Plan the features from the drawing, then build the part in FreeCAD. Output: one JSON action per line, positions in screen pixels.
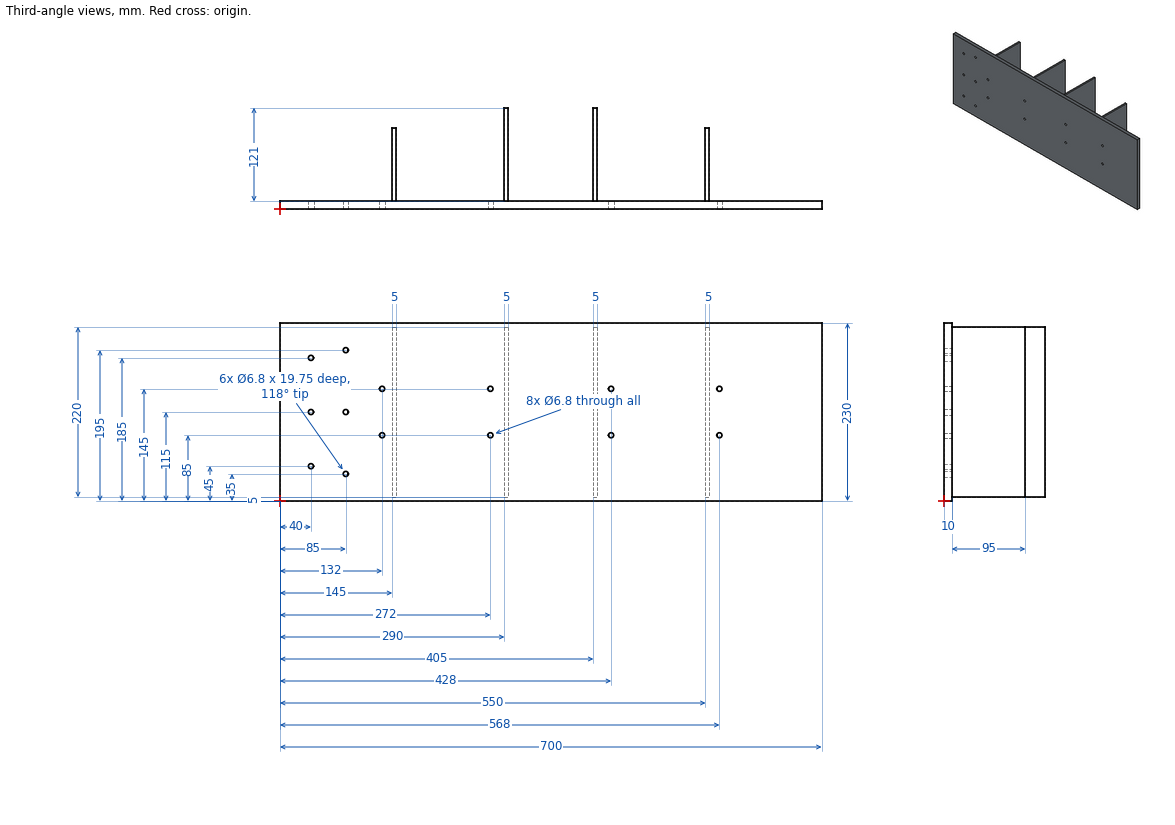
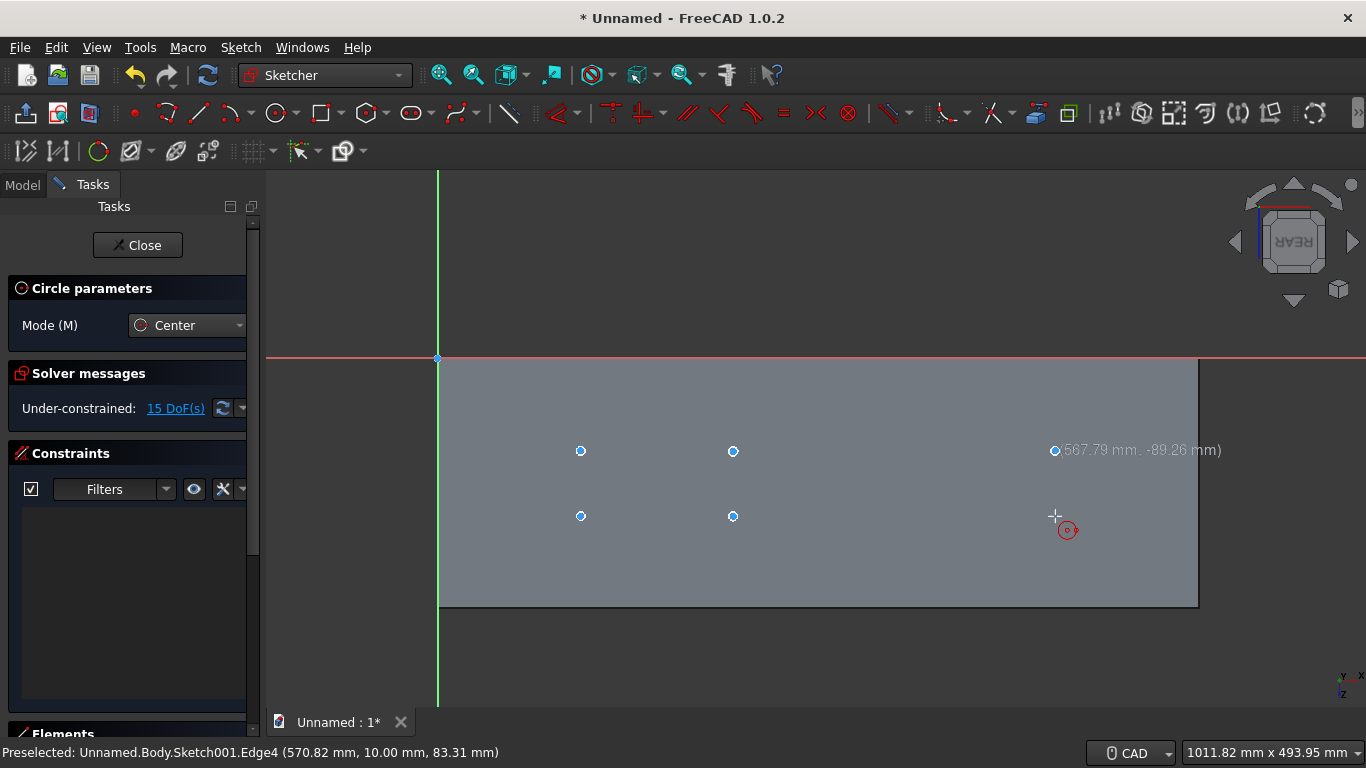
{"action": "left_click", "coordinate": [1055, 516]}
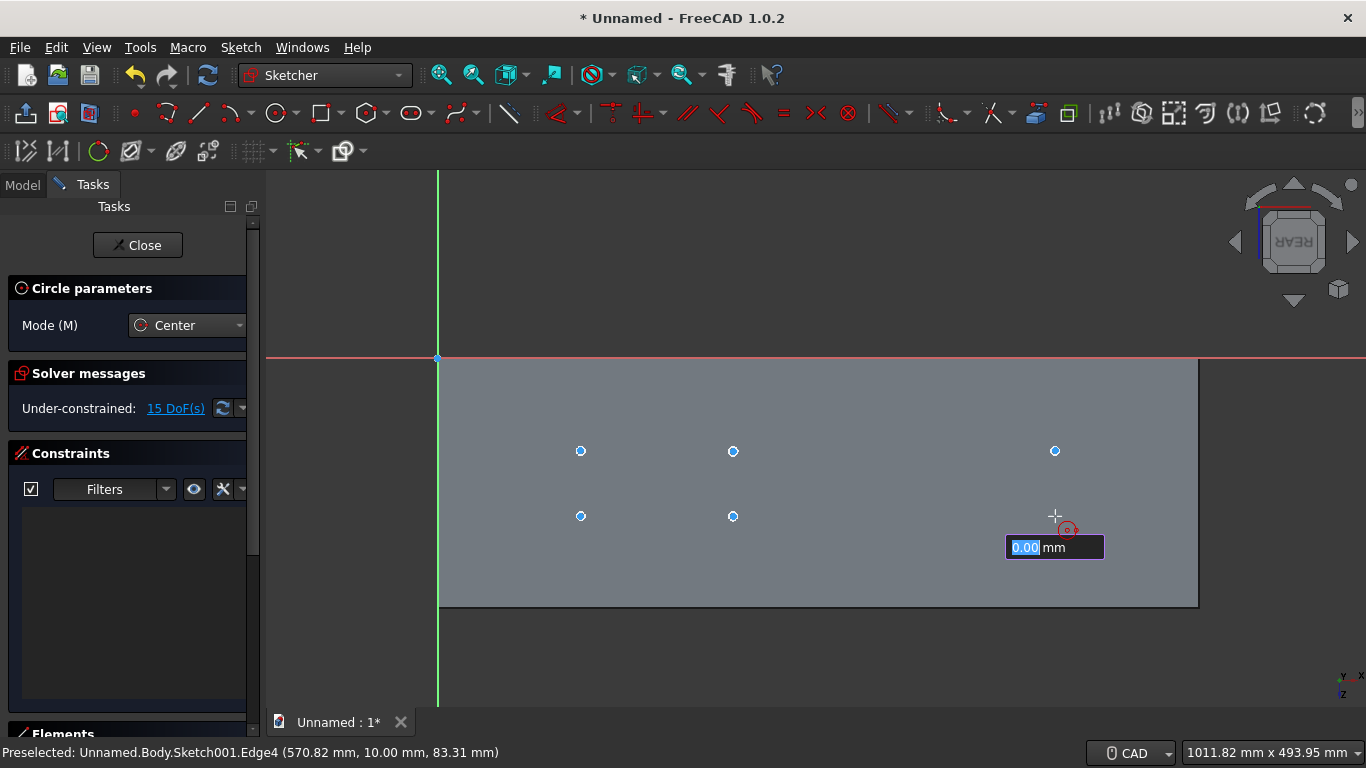
{"action": "scroll", "coordinate": [1058, 513], "scroll_direction": "up", "scroll_amount": 8}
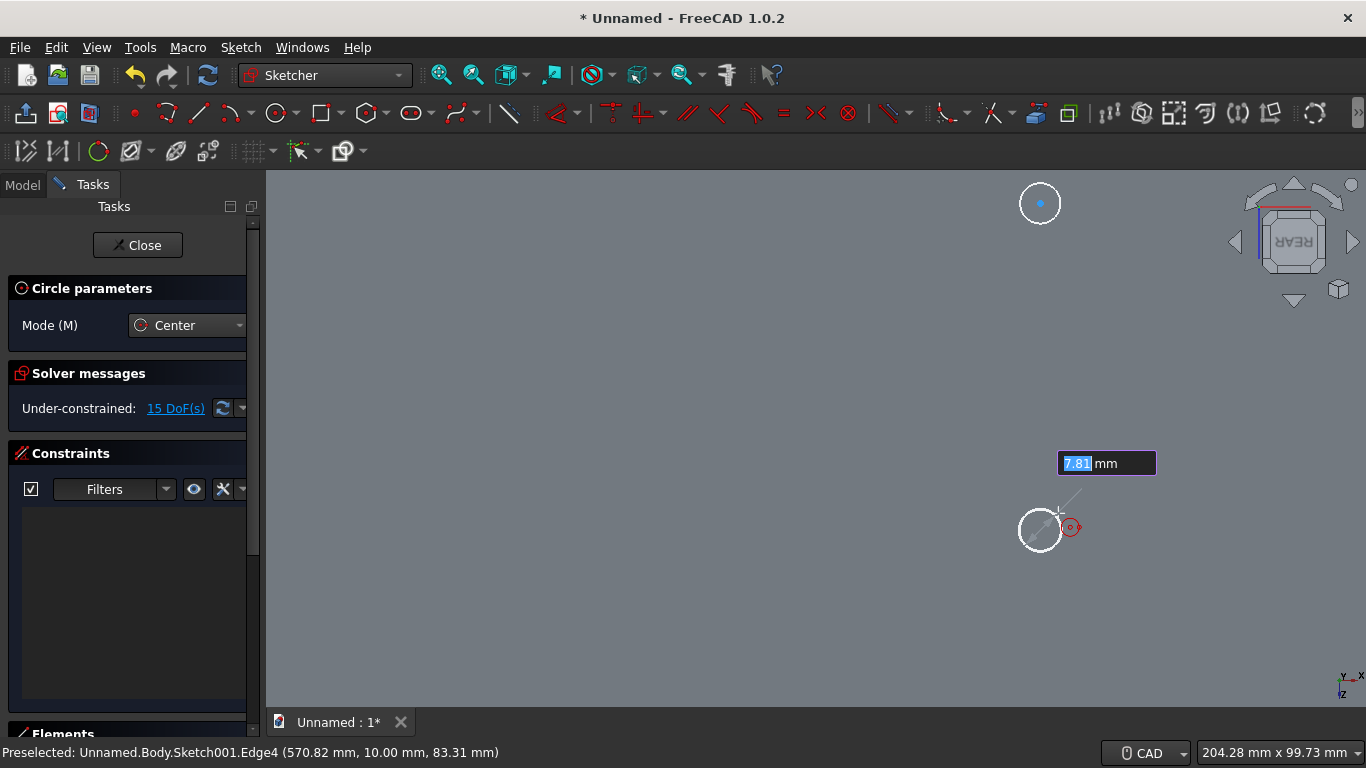
{"action": "left_click", "coordinate": [1054, 511]}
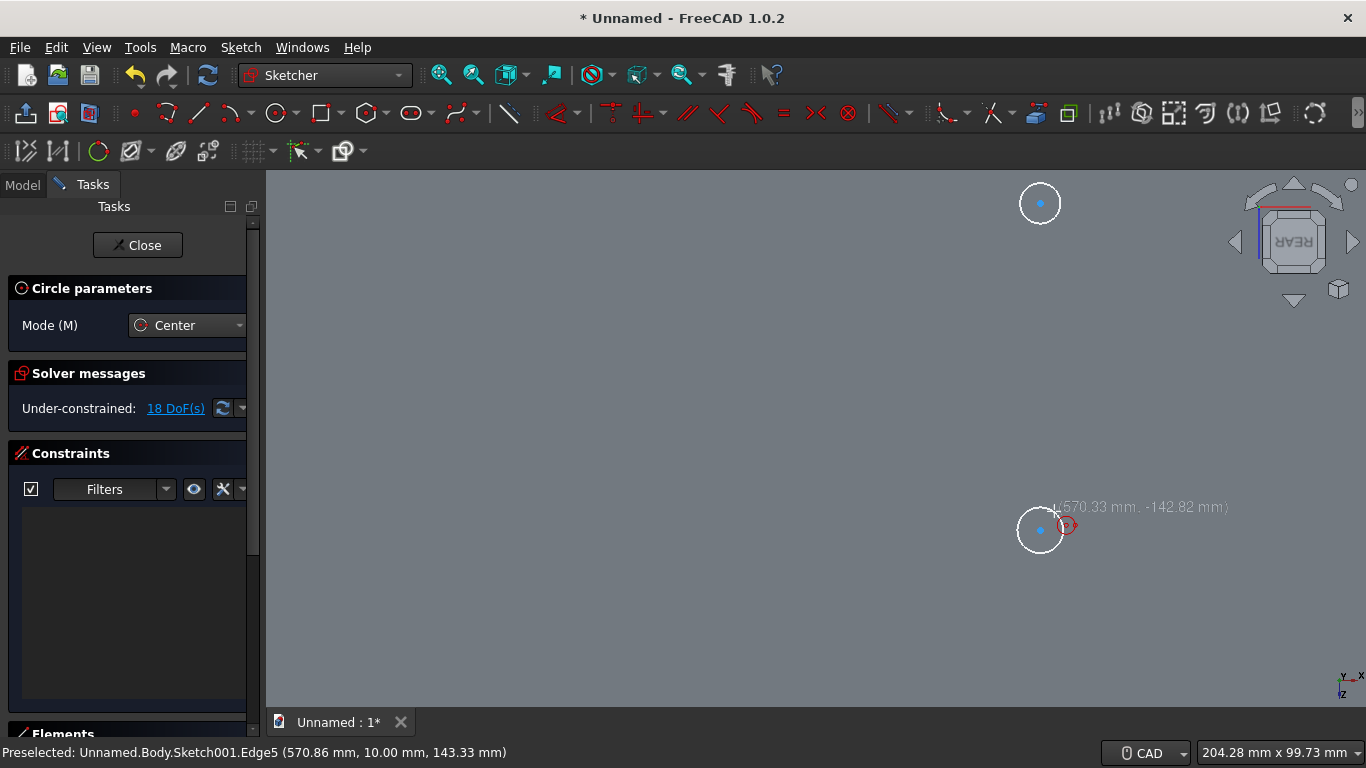
{"action": "scroll", "coordinate": [1058, 513], "scroll_direction": "down", "scroll_amount": 8}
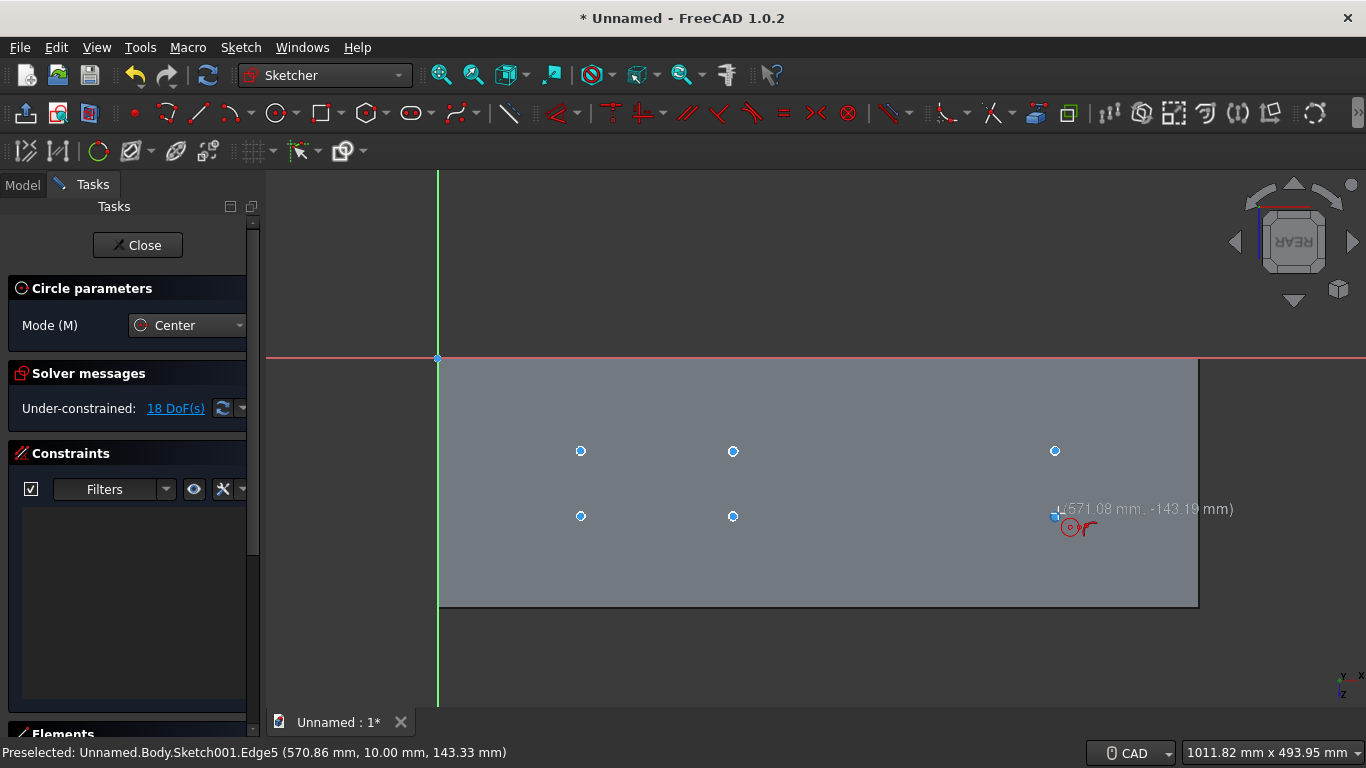
{"action": "scroll", "coordinate": [903, 516], "scroll_direction": "up", "scroll_amount": 10}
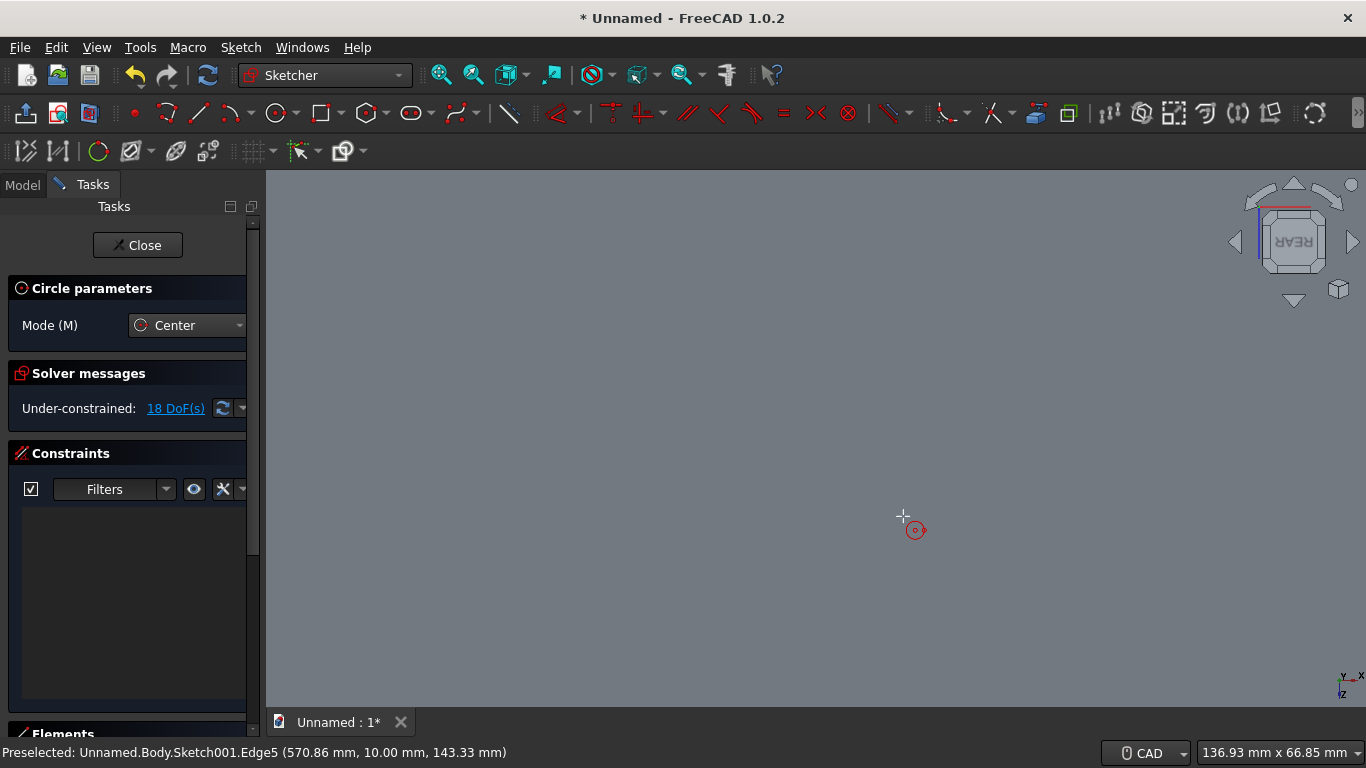
{"action": "scroll", "coordinate": [903, 516], "scroll_direction": "down", "scroll_amount": 10}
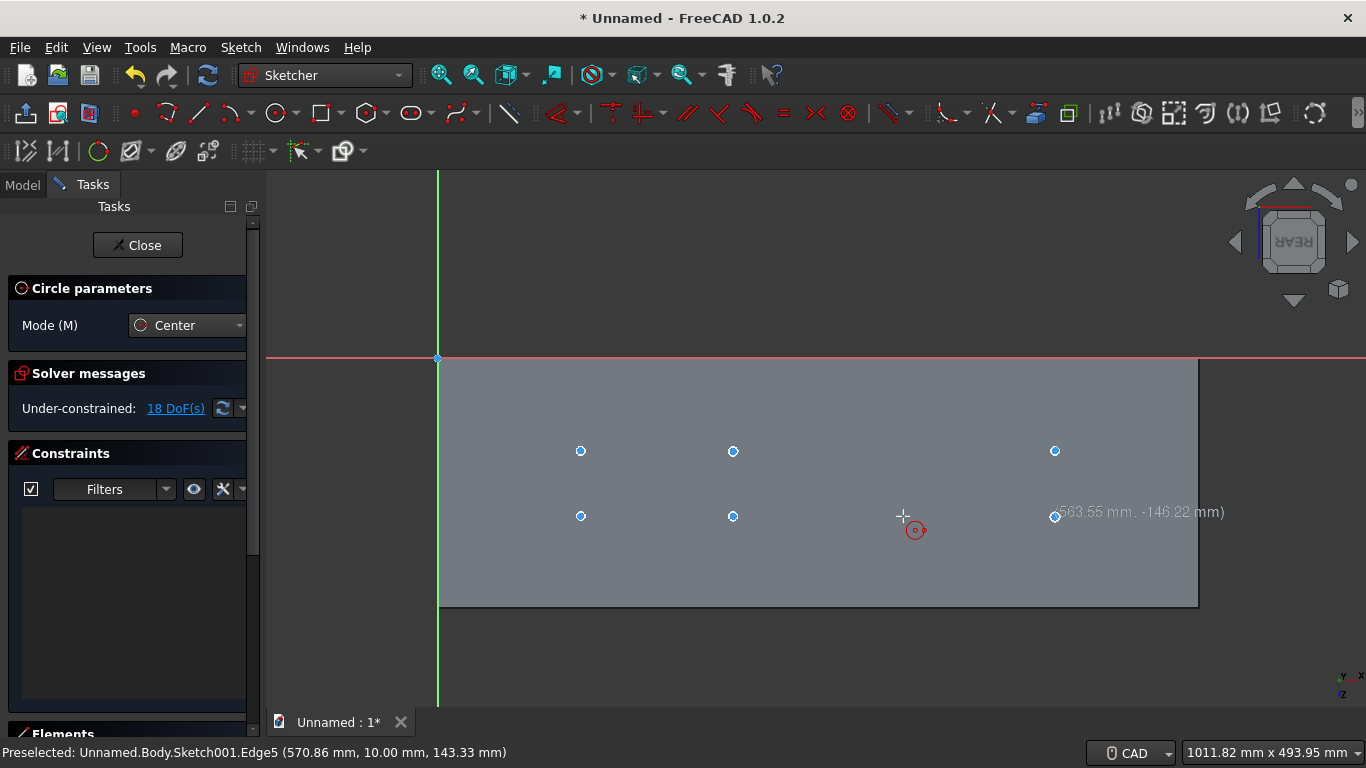
{"action": "left_click", "coordinate": [903, 516]}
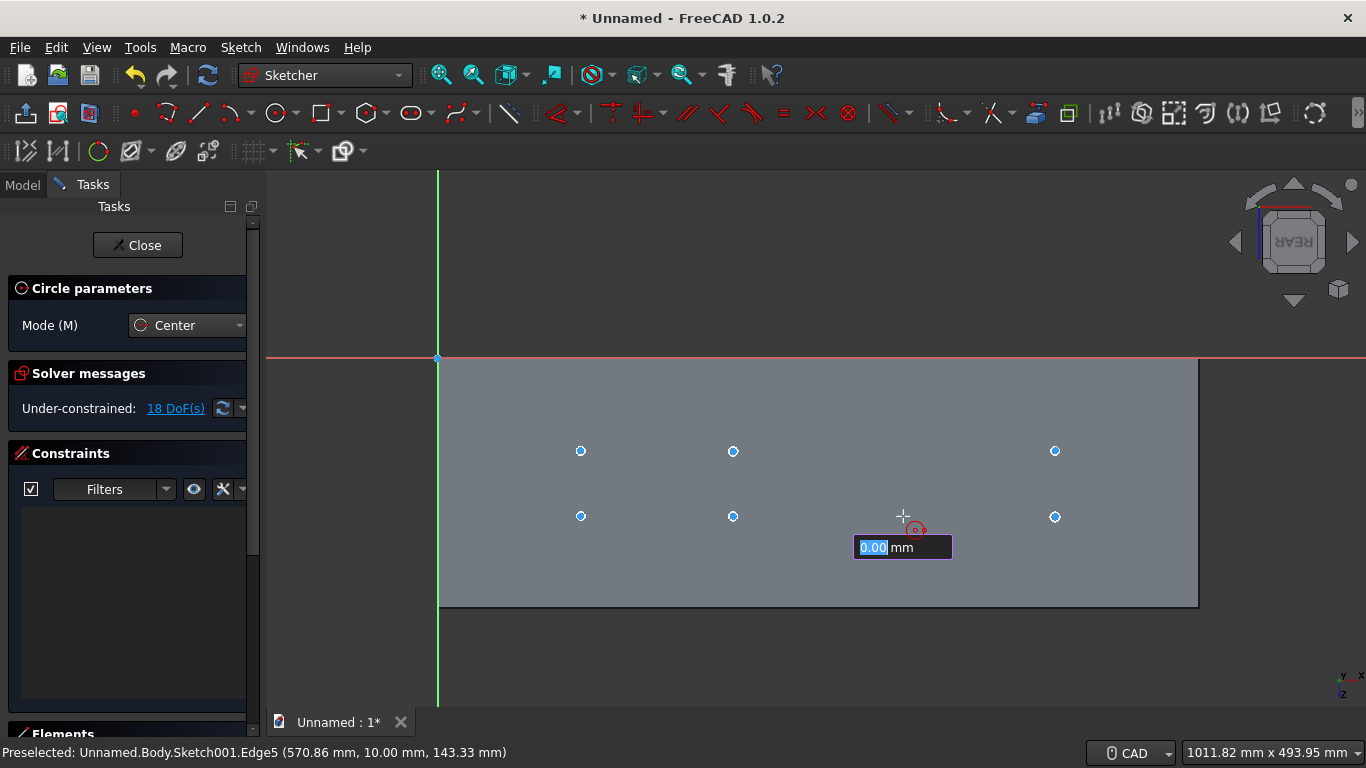
{"action": "scroll", "coordinate": [906, 513], "scroll_direction": "up", "scroll_amount": 8}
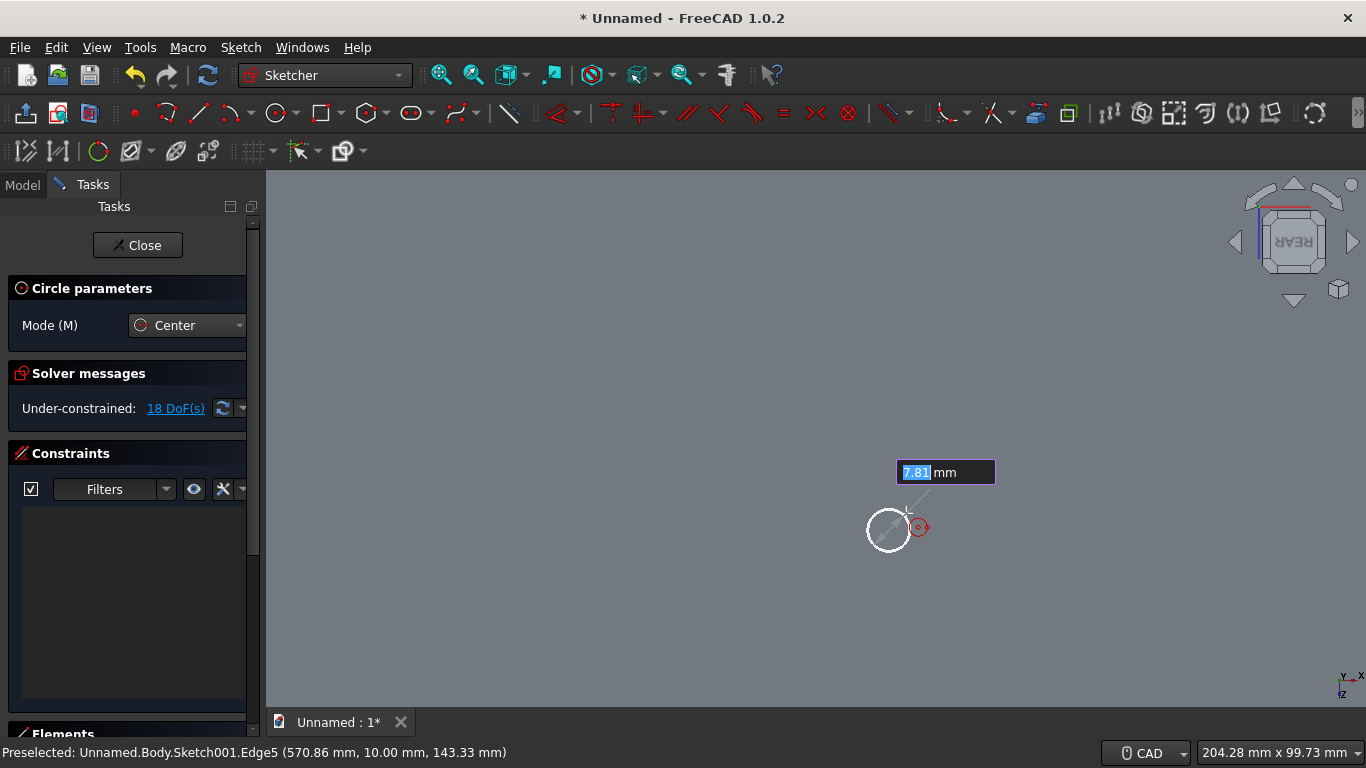
{"action": "left_click", "coordinate": [902, 511]}